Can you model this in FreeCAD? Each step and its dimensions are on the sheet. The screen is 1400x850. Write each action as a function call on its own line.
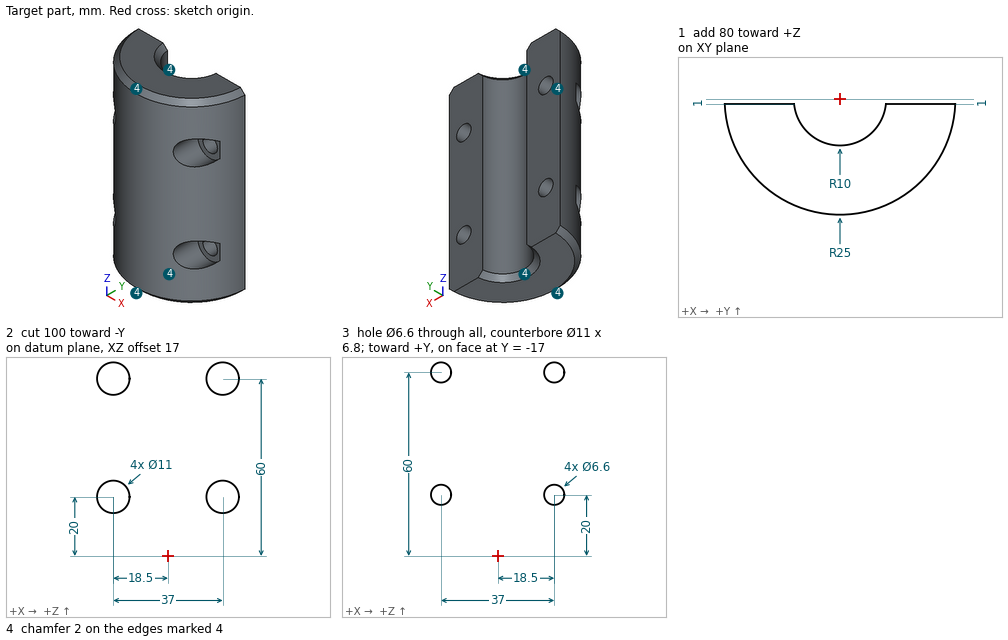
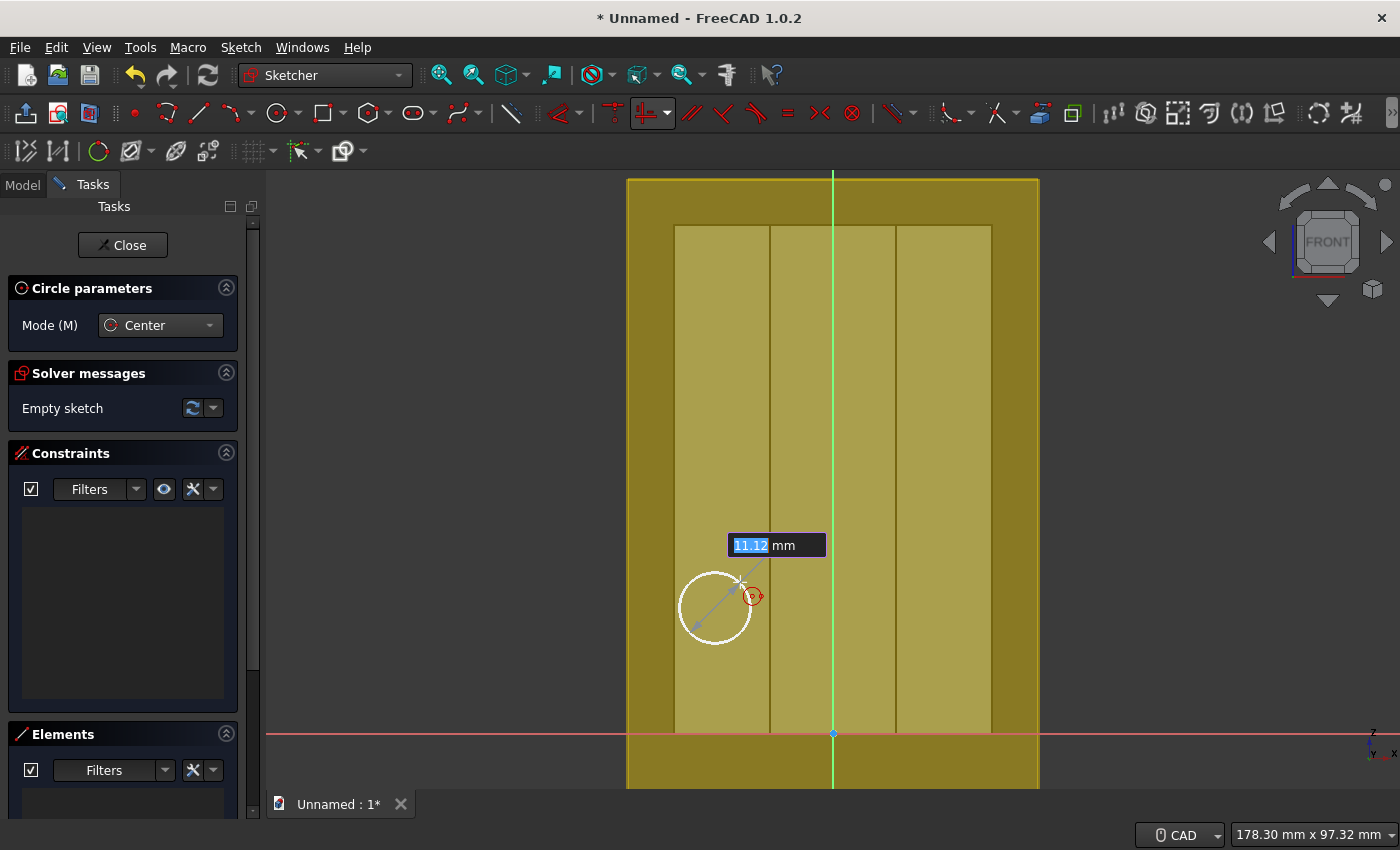
text(11)
key(Return)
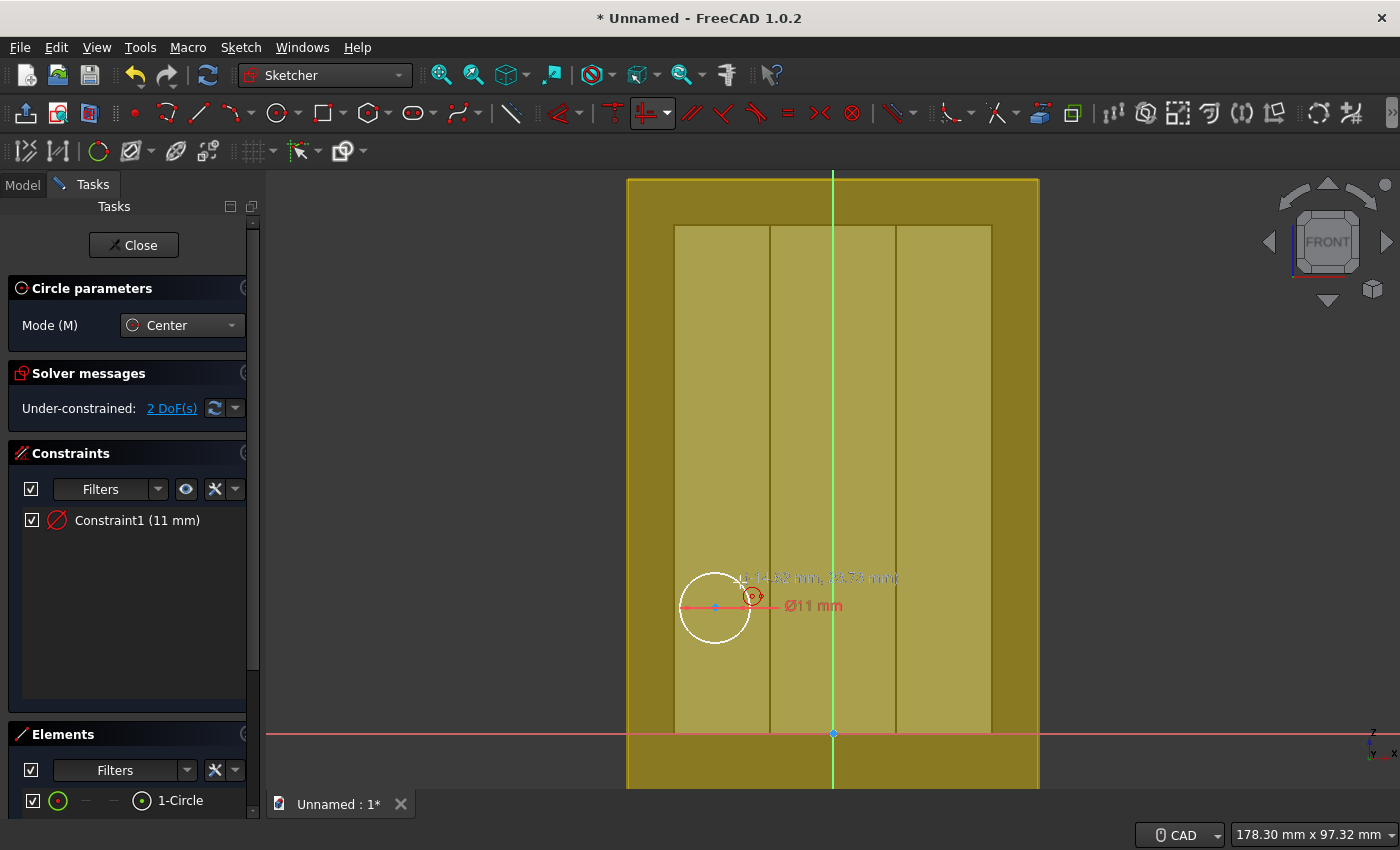
click(951, 607)
move(975, 582)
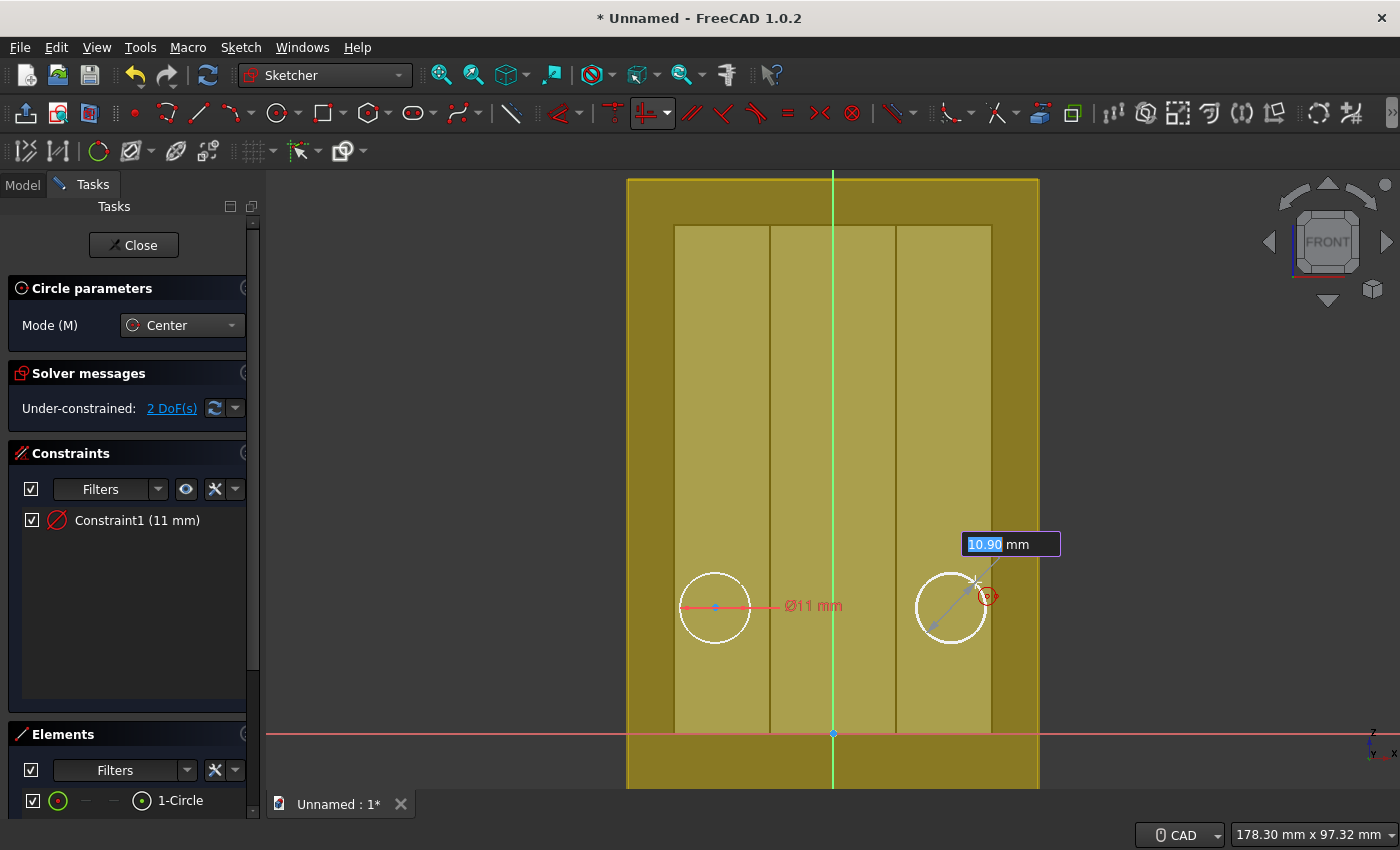
text(11)
key(Return)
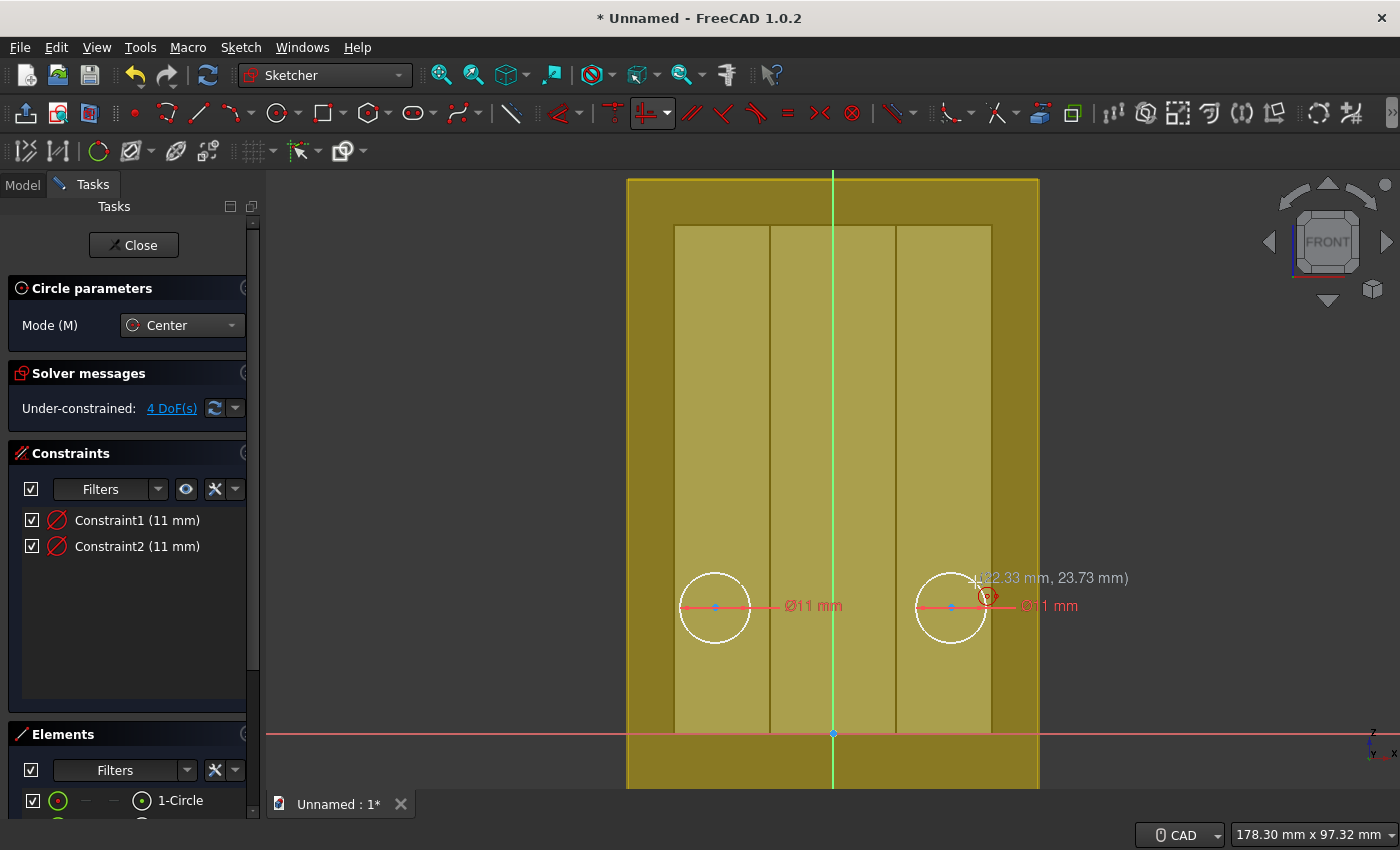
click(951, 352)
move(975, 328)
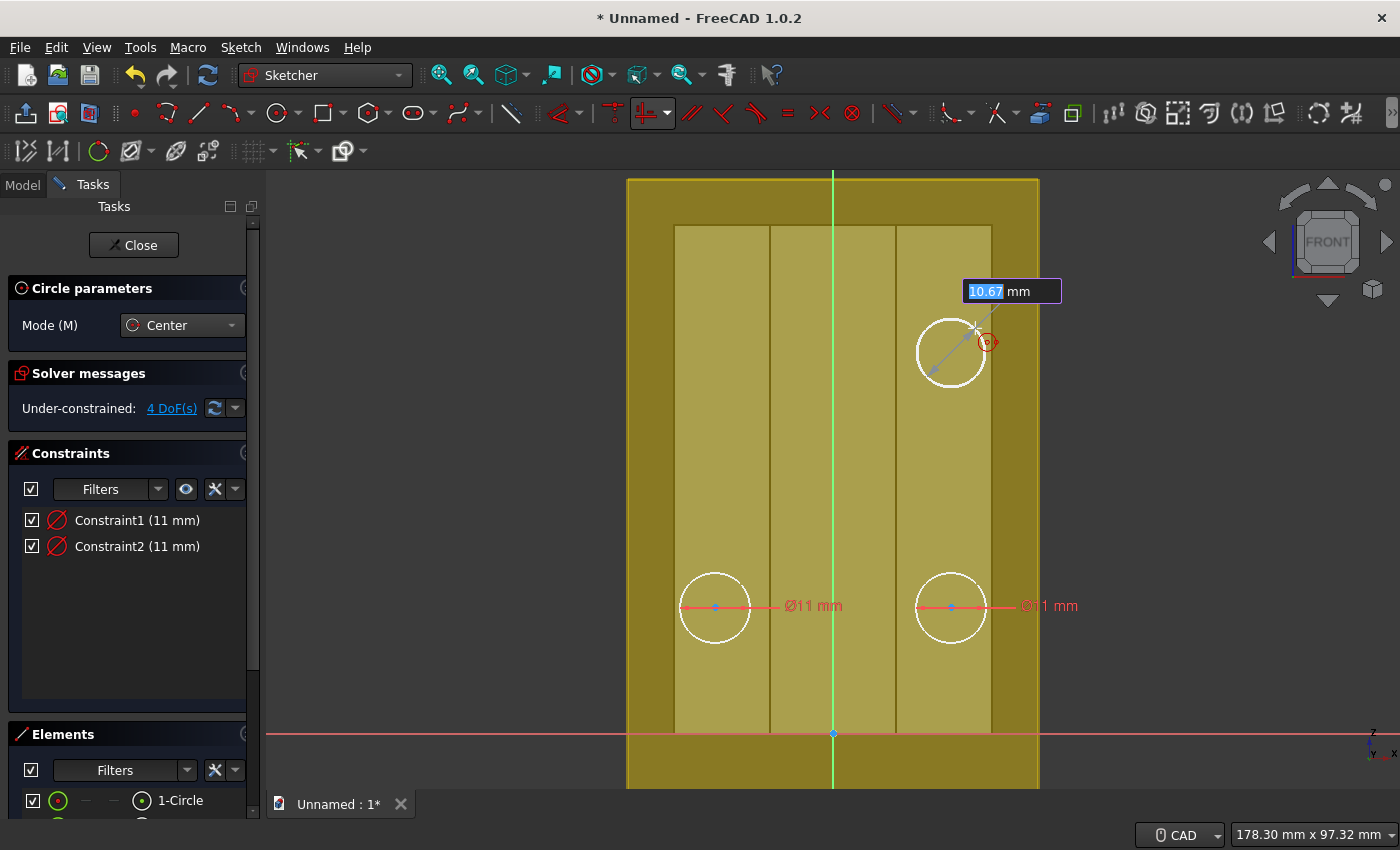
text(11)
key(Return)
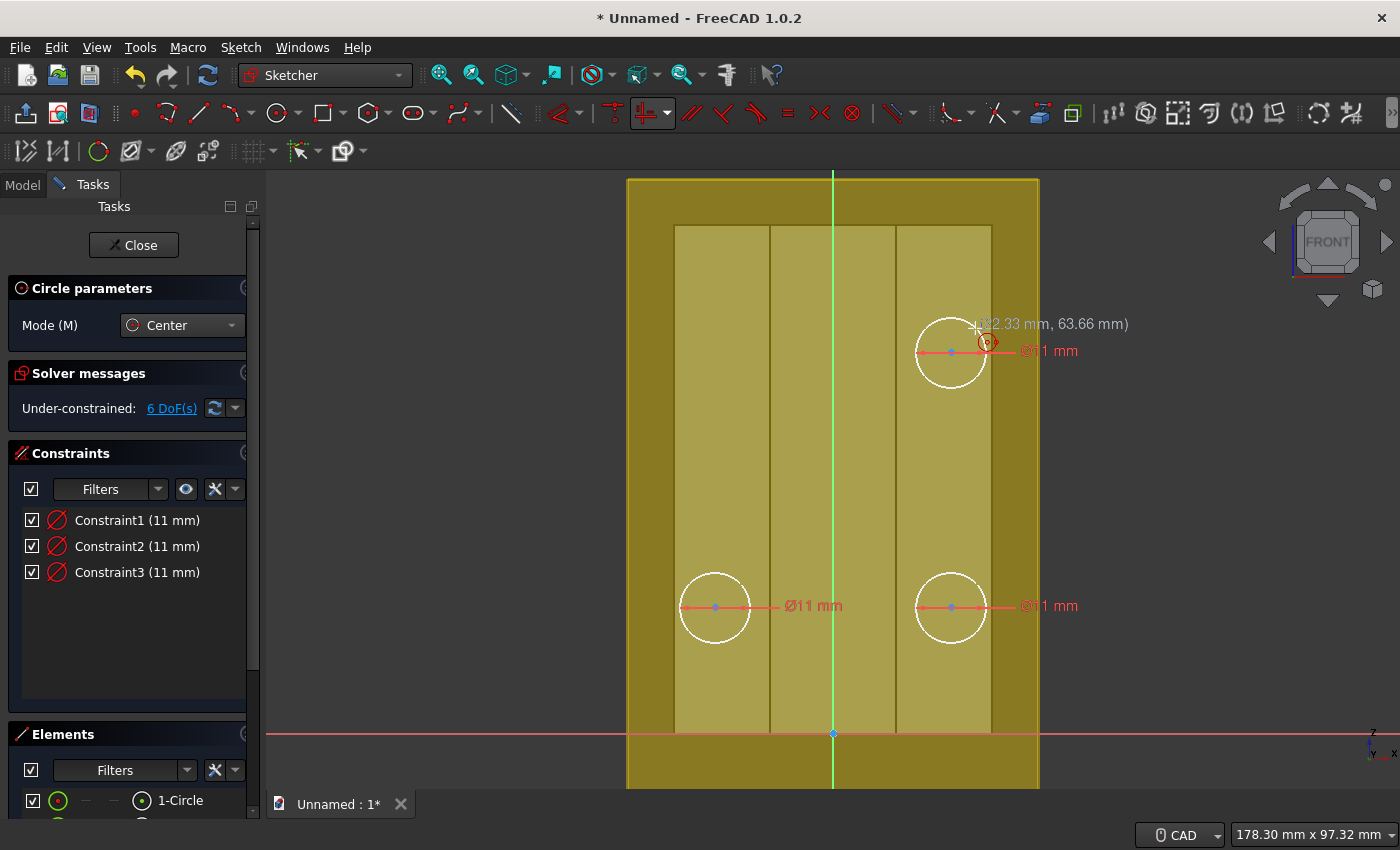
click(715, 352)
move(740, 328)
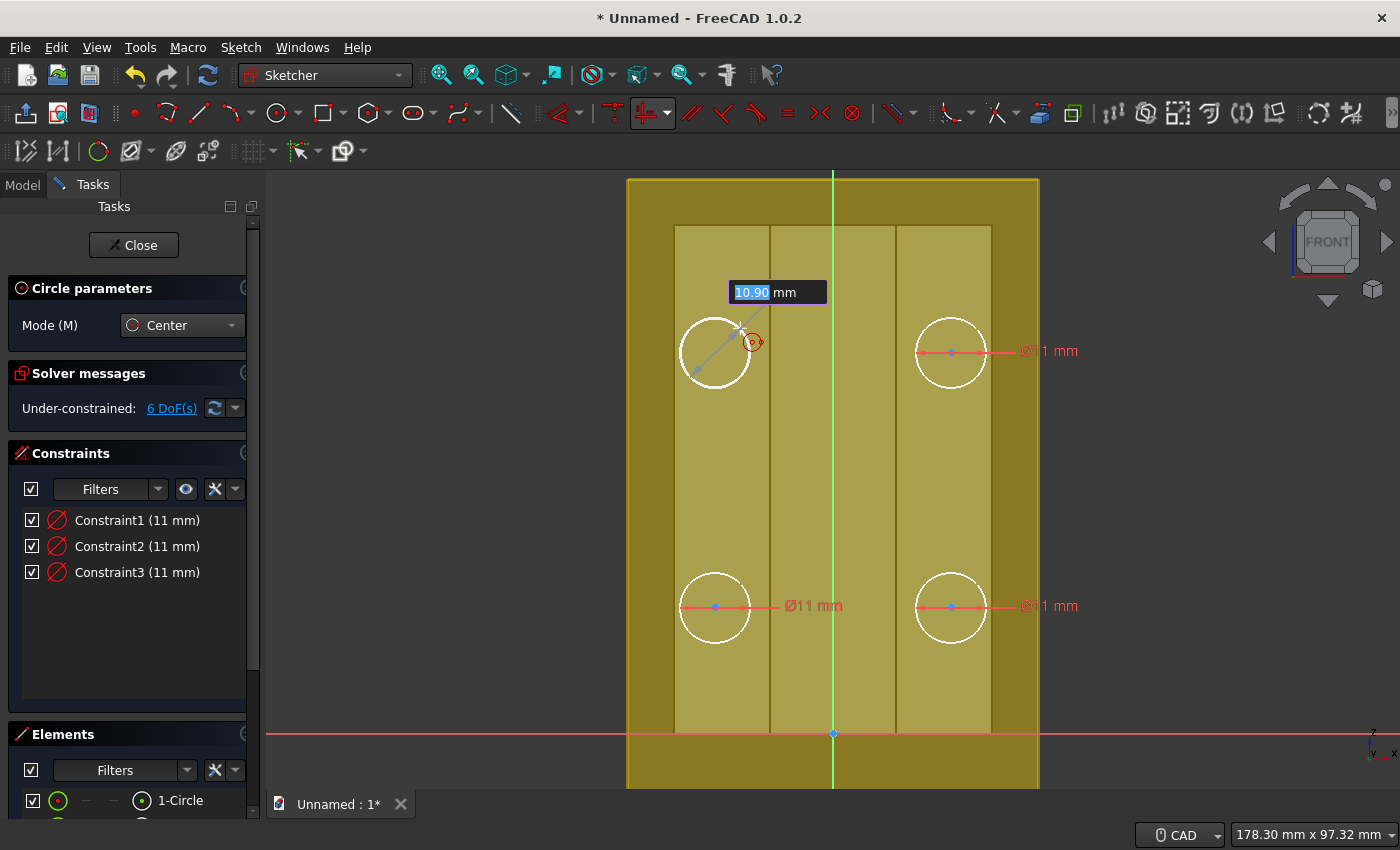
text(11)
key(Return)
key(Escape)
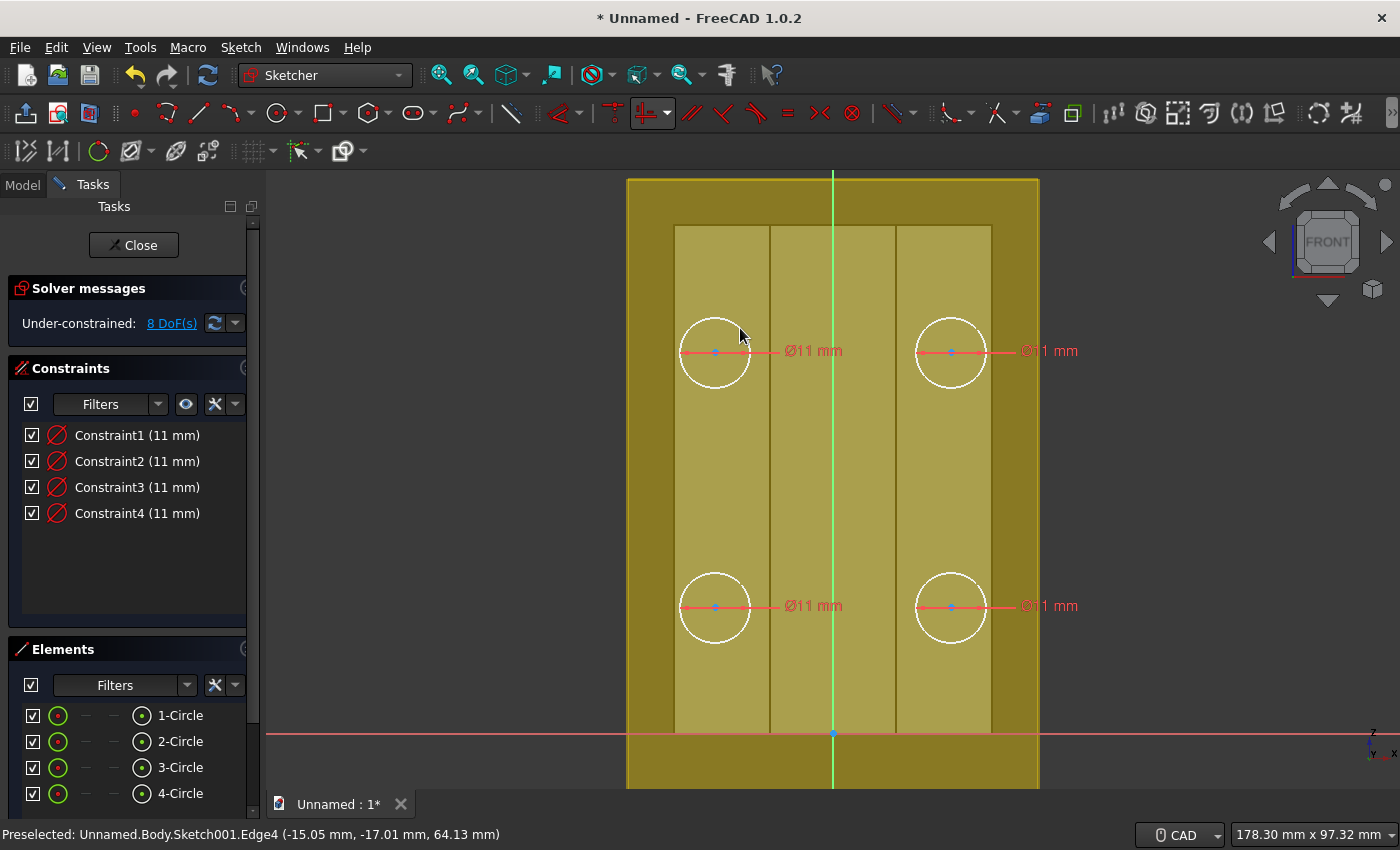
click(715, 608)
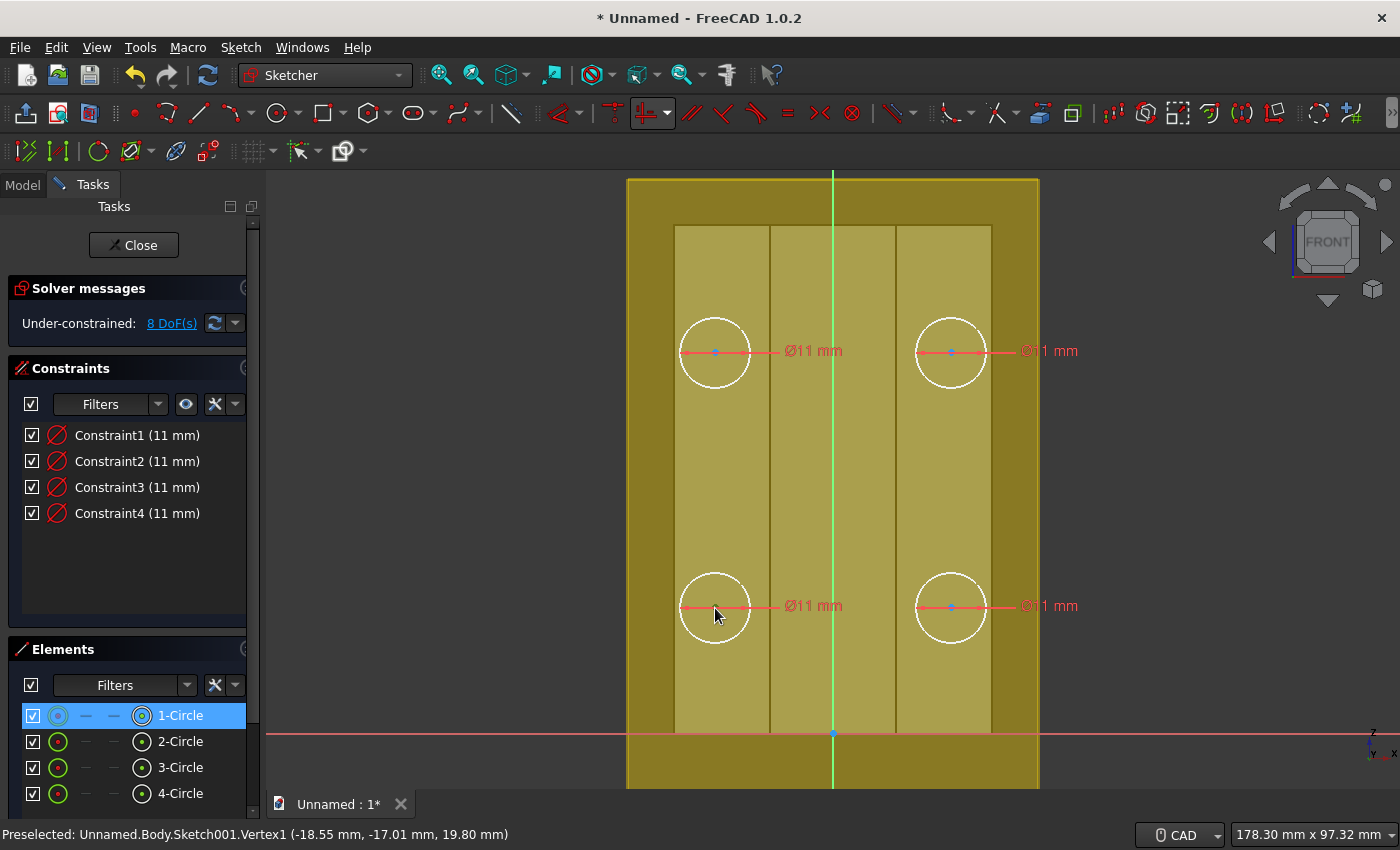
click(951, 608)